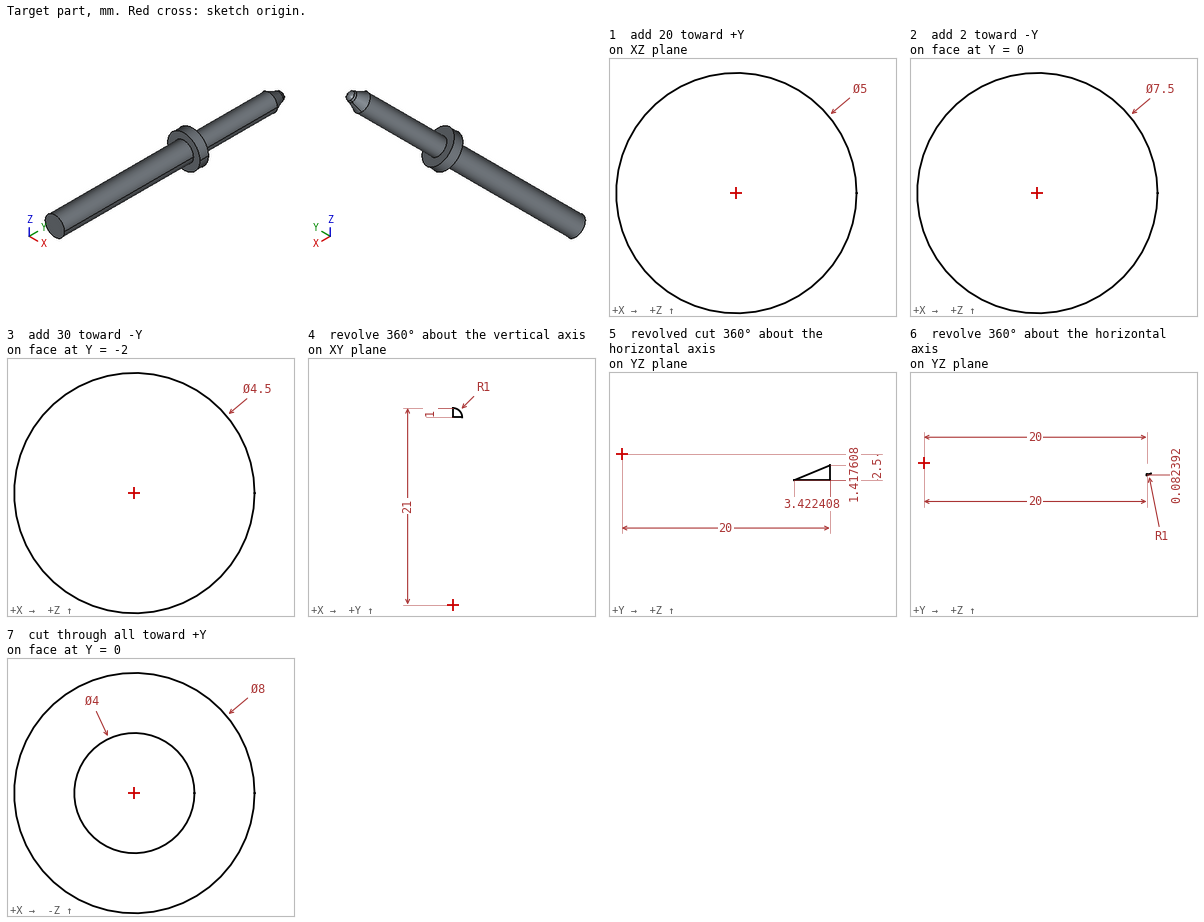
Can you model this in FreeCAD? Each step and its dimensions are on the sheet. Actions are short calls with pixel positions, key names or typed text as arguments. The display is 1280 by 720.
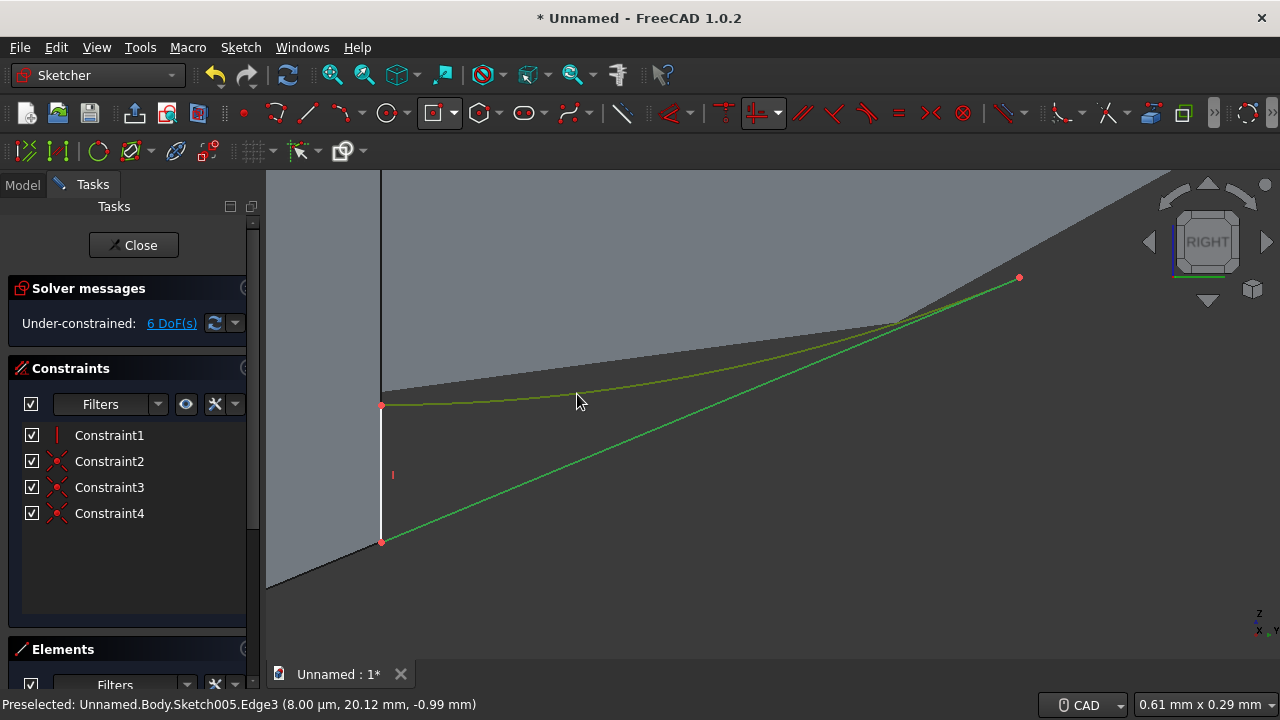
key(t)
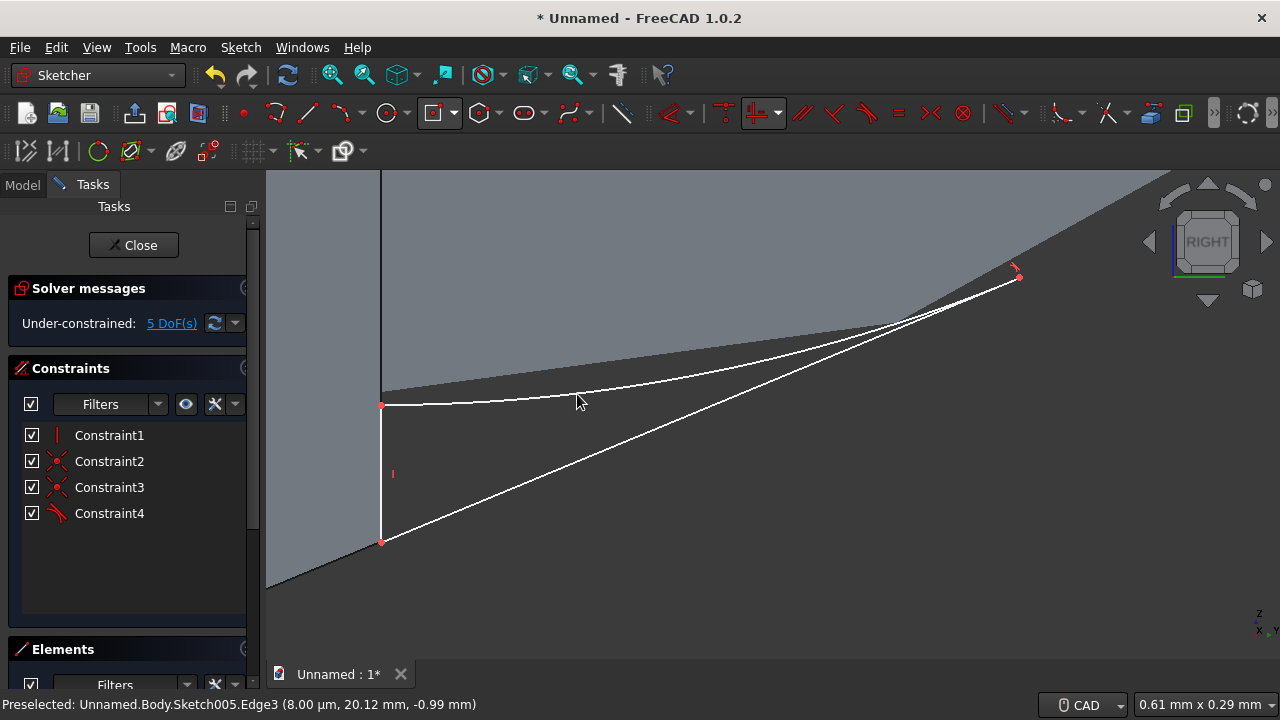
scroll(705, 568, down, 9)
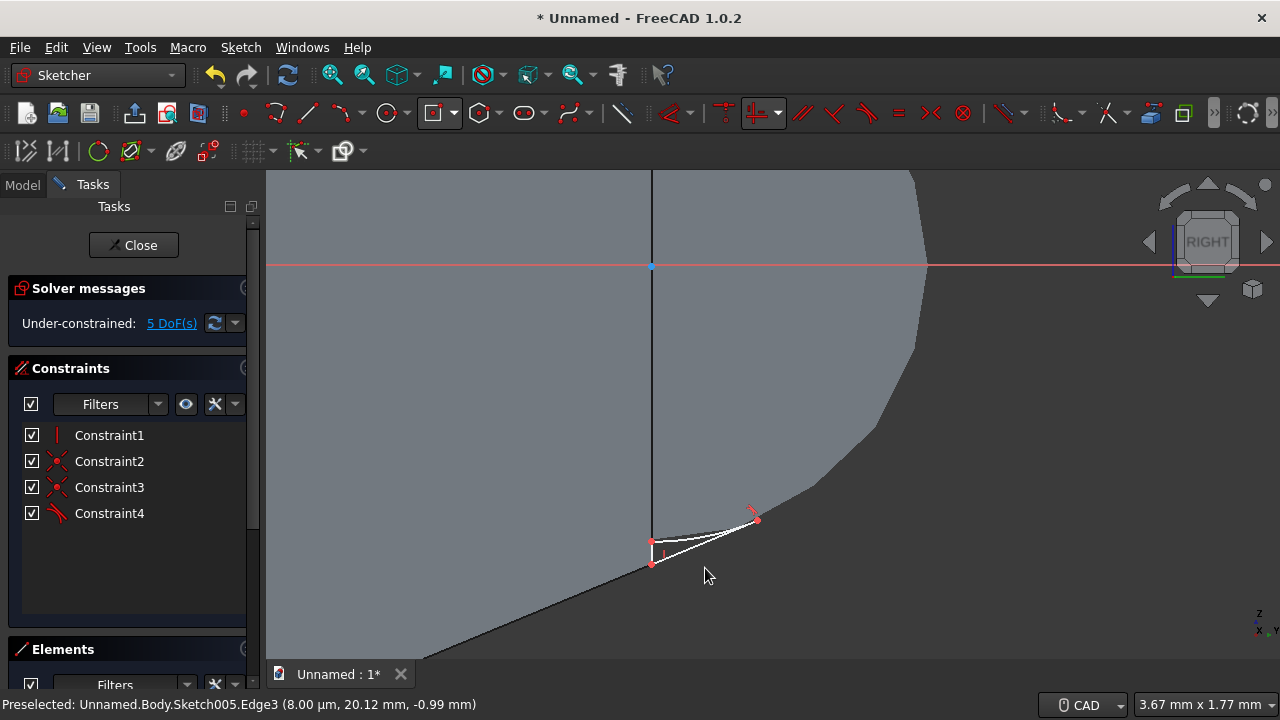
click(652, 266)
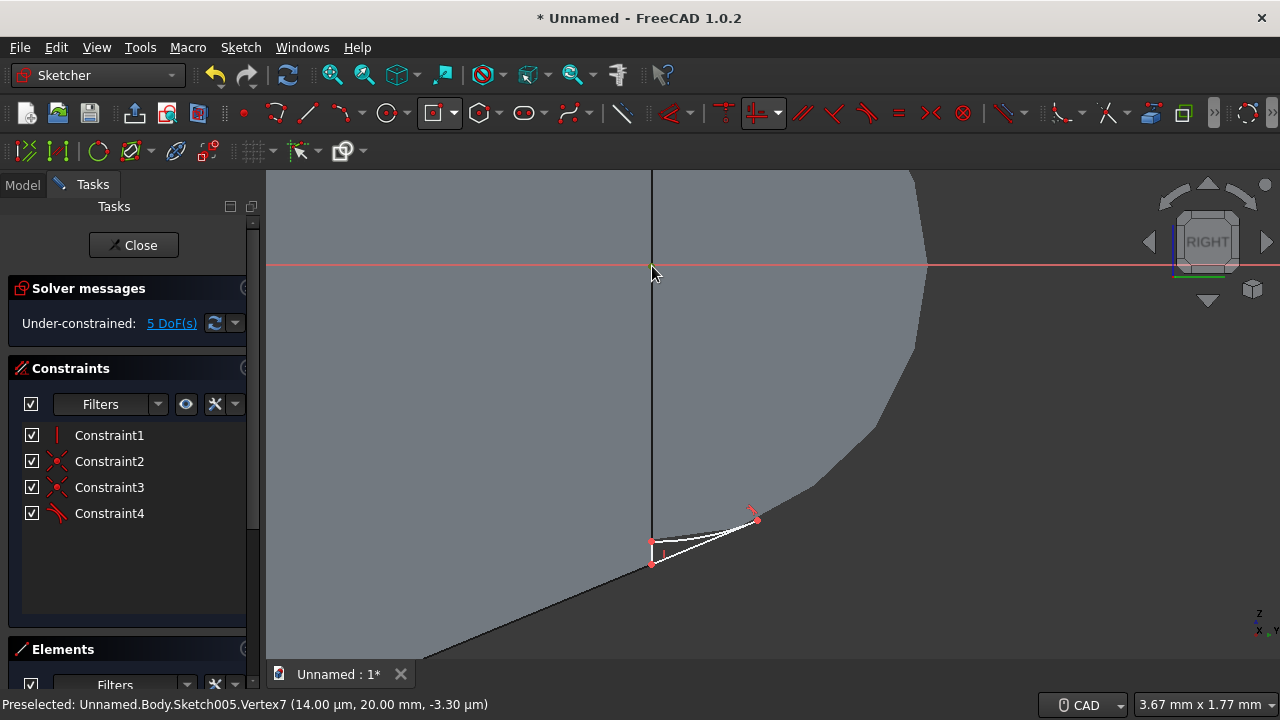
click(353, 265)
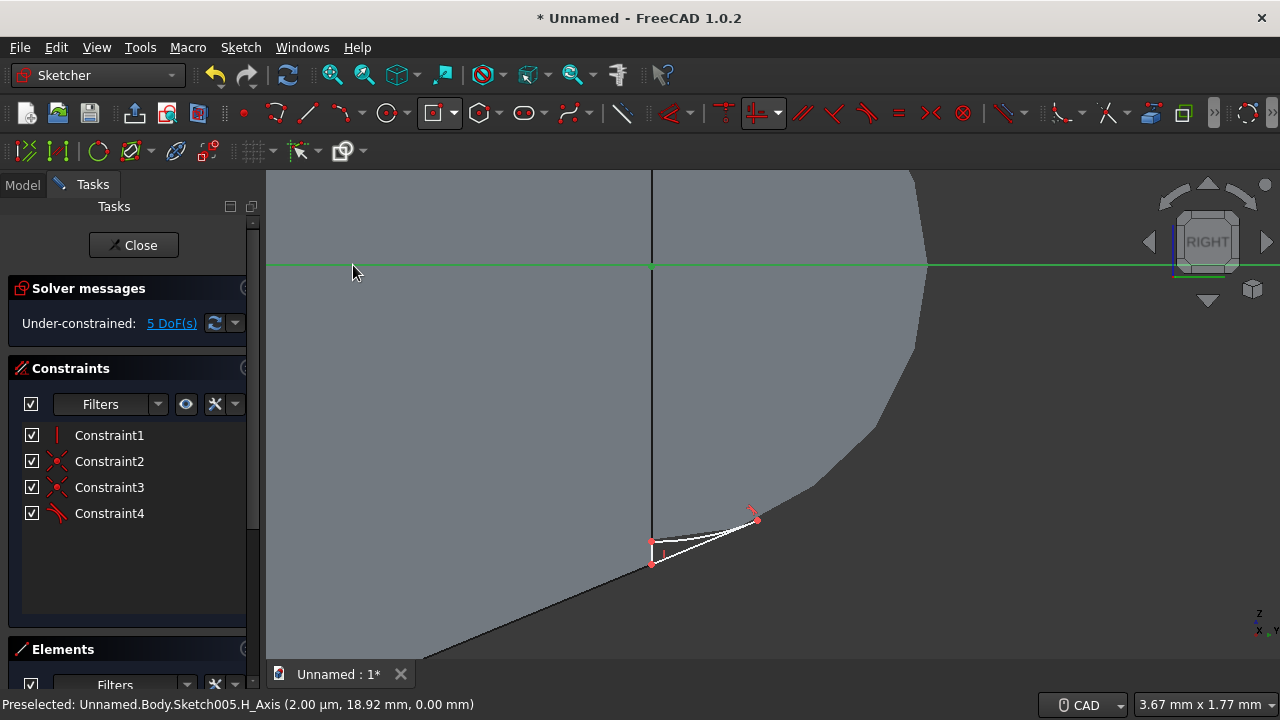
click(724, 114)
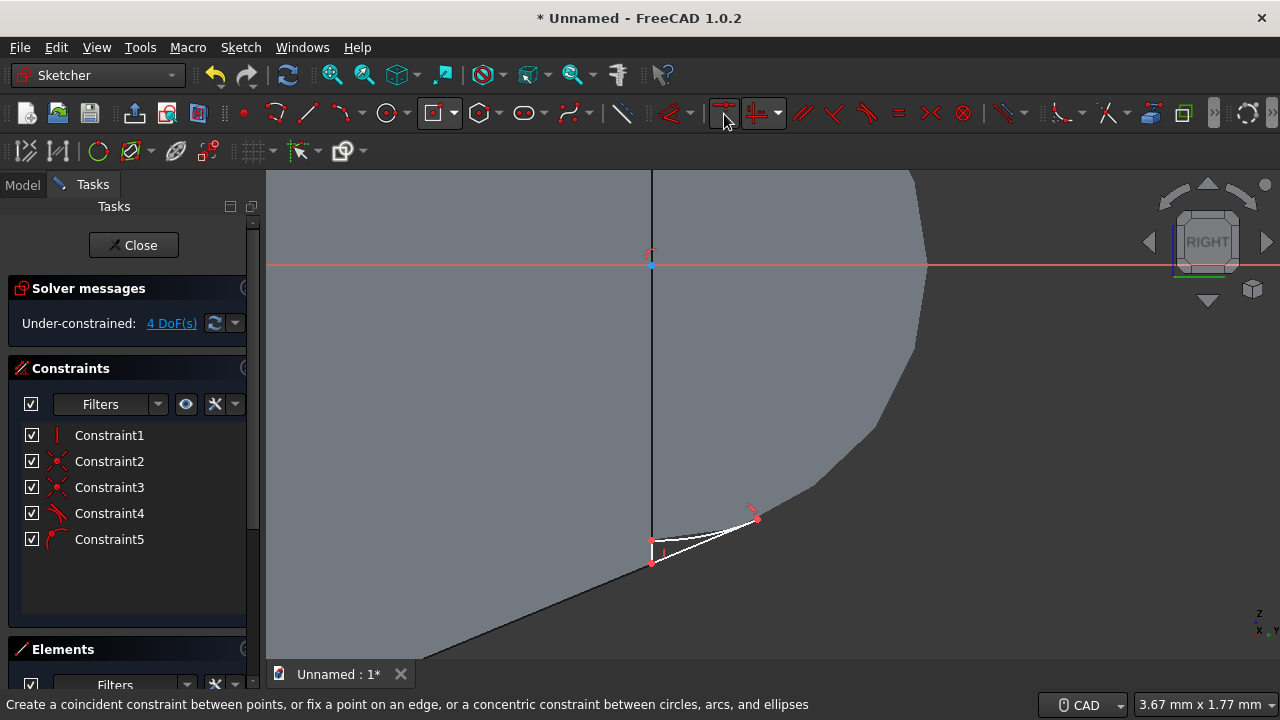
click(670, 114)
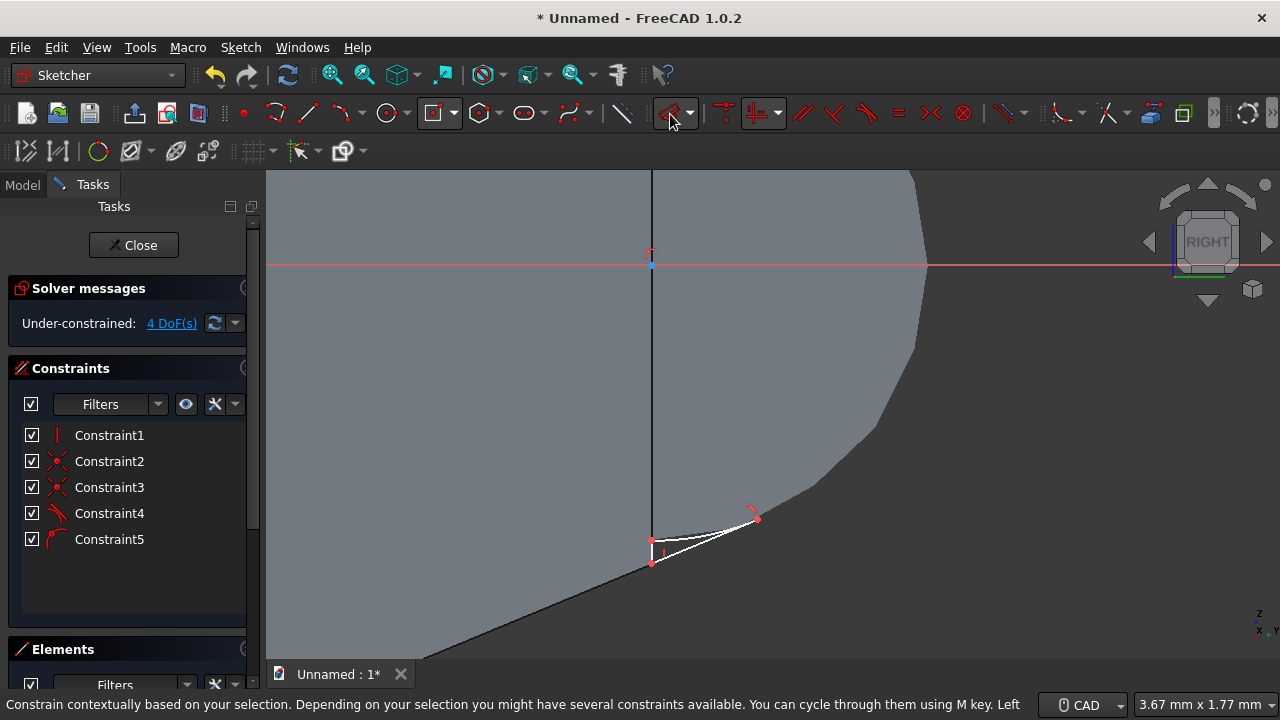
scroll(684, 539, up, 2)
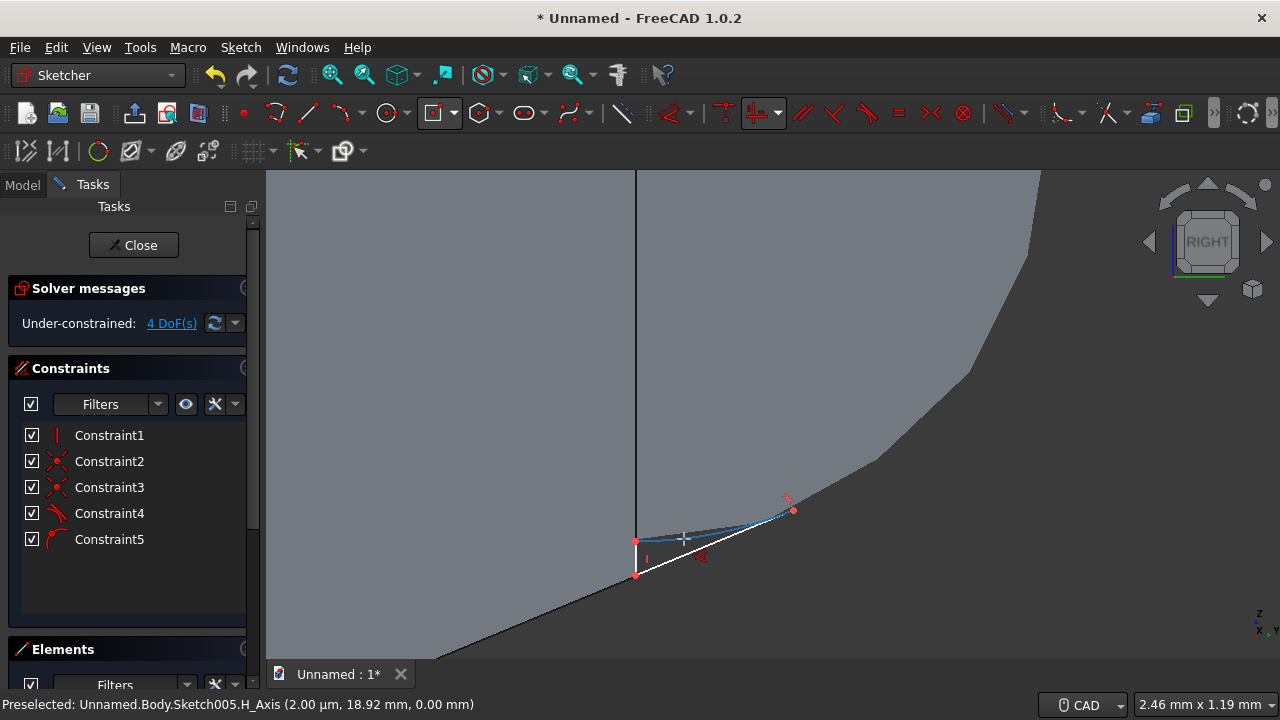
click(684, 539)
click(688, 571)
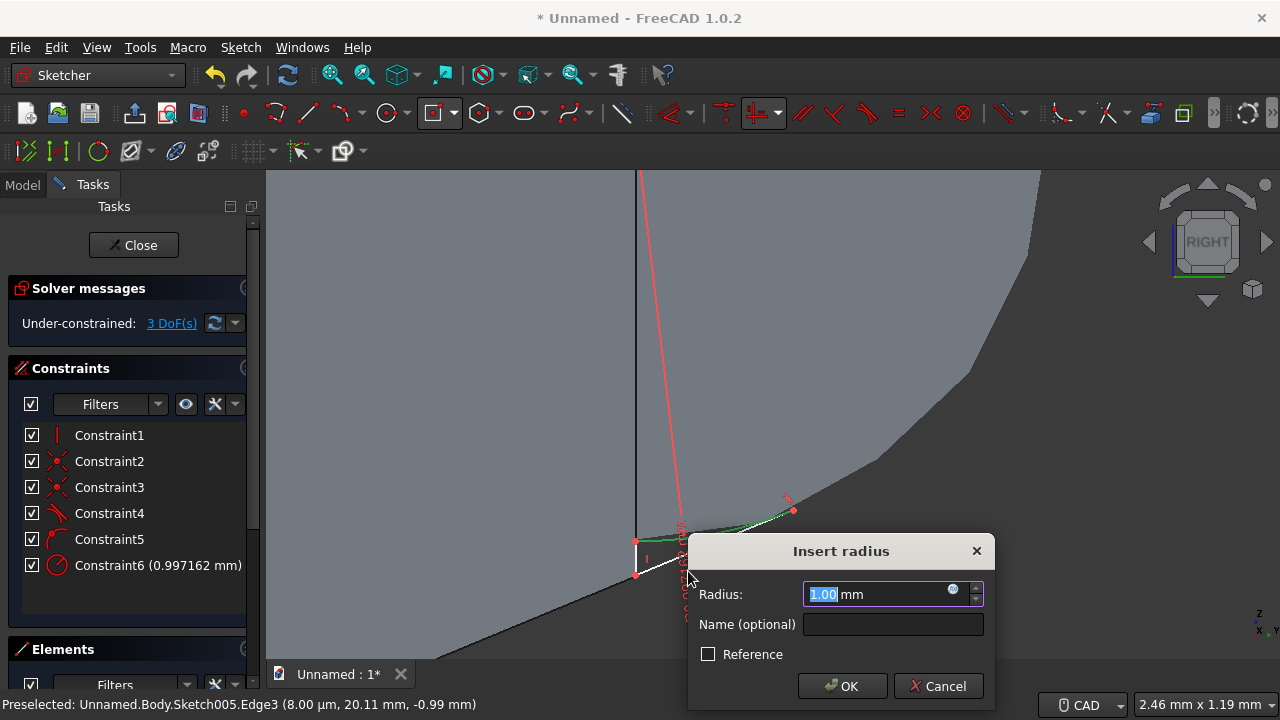
text(1)
key(Return)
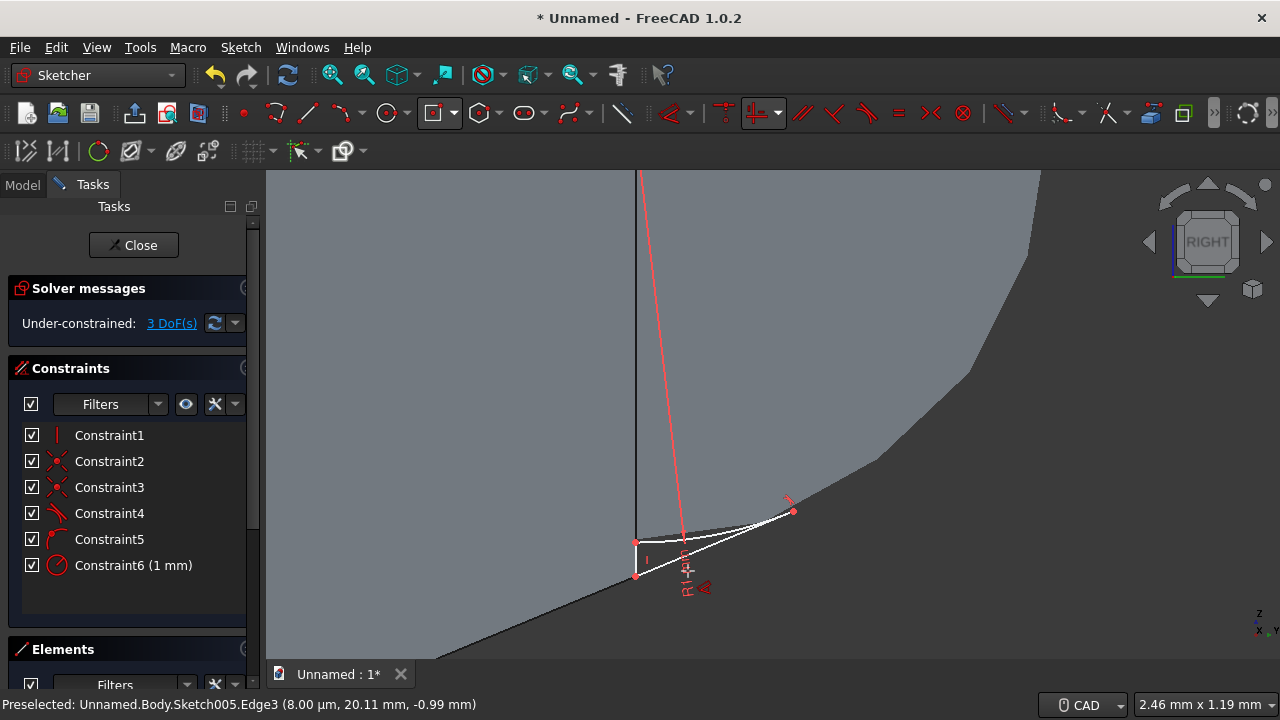
click(636, 543)
click(465, 577)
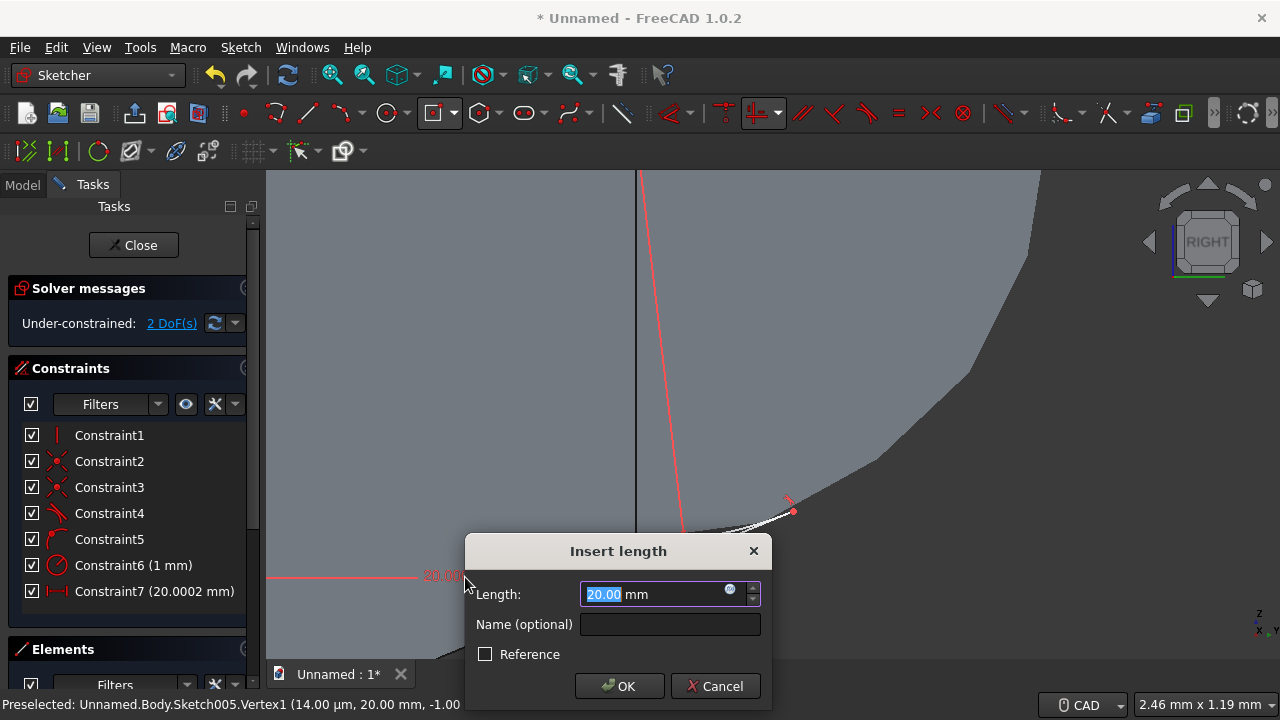
text(20)
key(Return)